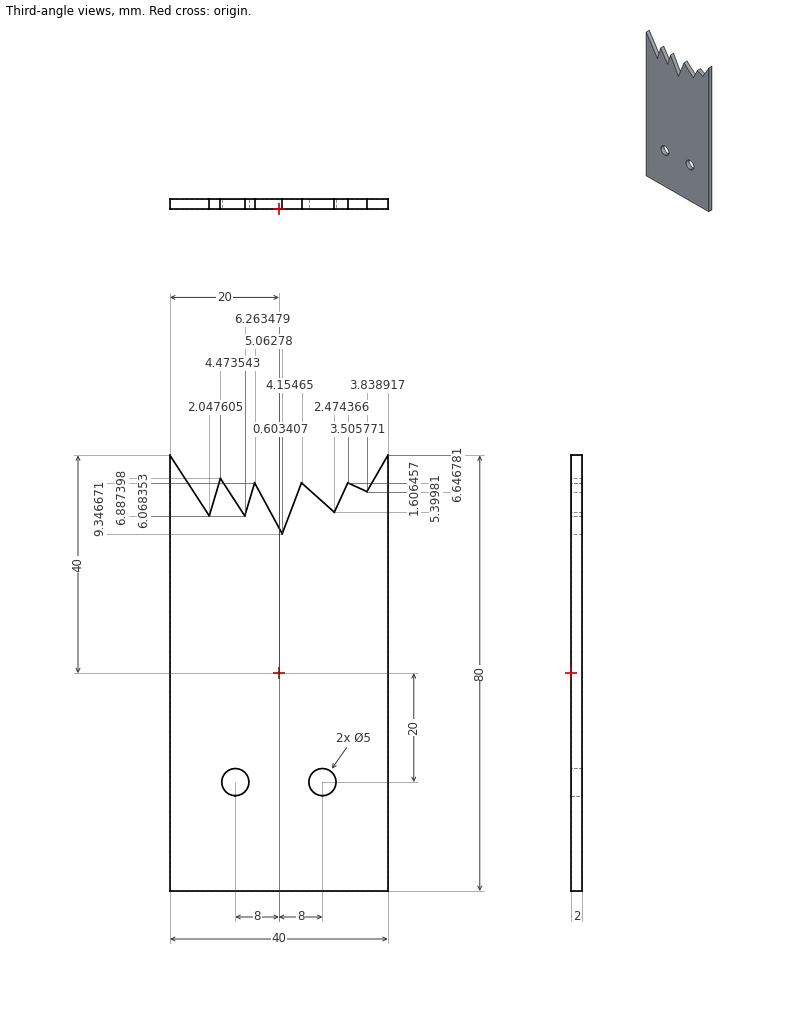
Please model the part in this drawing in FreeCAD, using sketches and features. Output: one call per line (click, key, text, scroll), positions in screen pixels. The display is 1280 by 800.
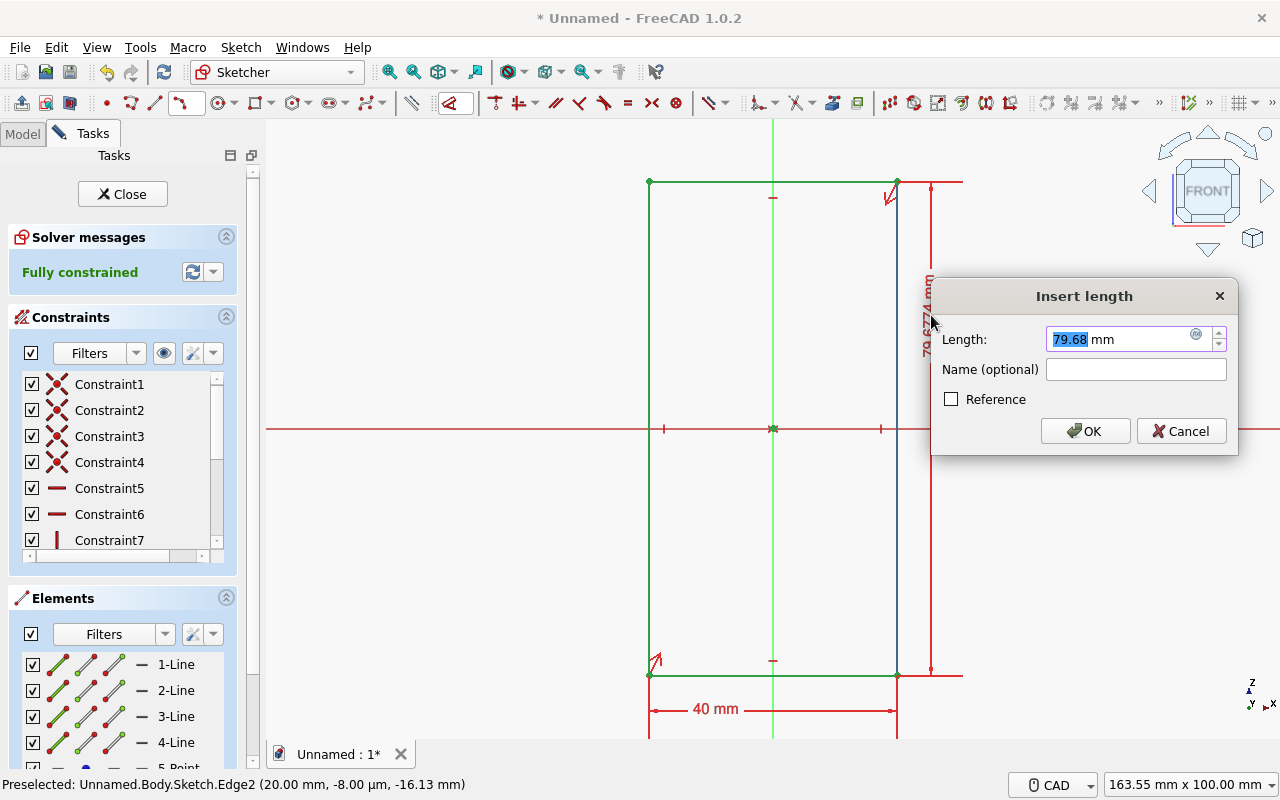
text(80)
key(Return)
key(Escape)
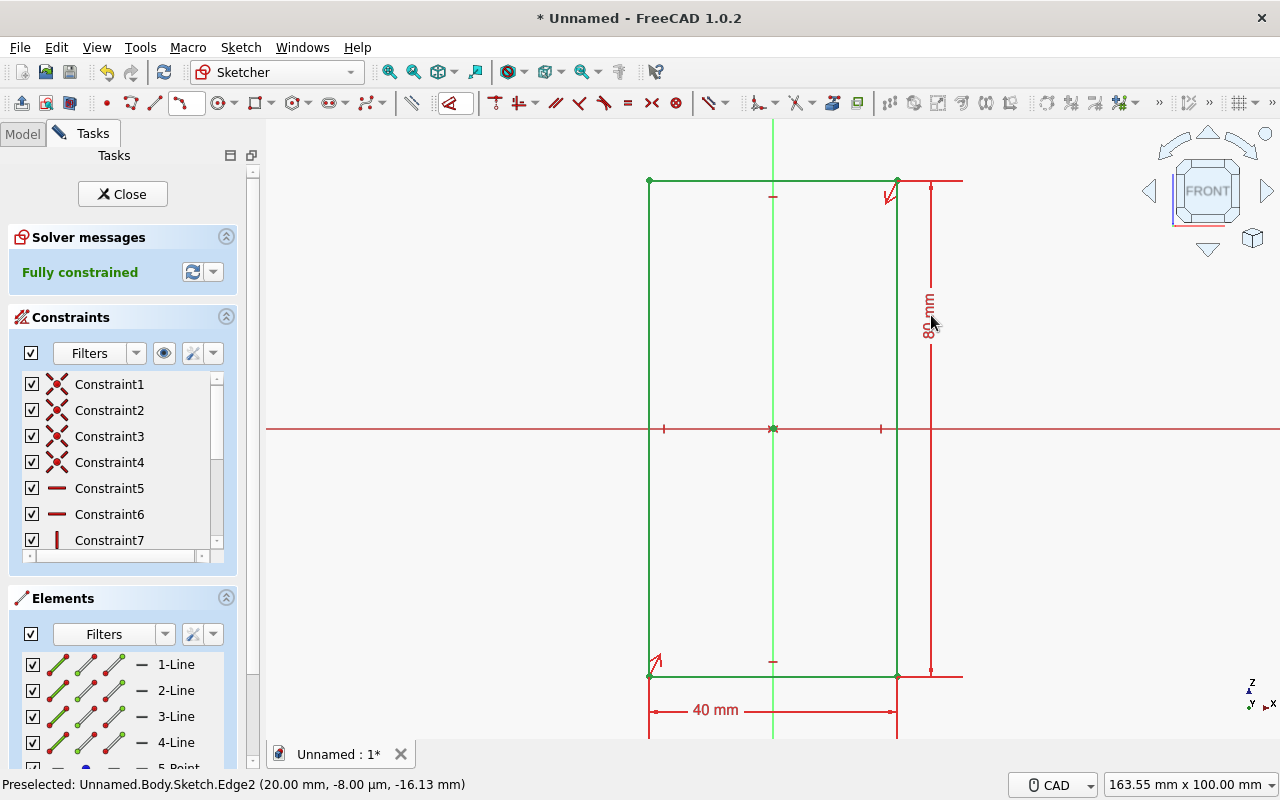
click(123, 194)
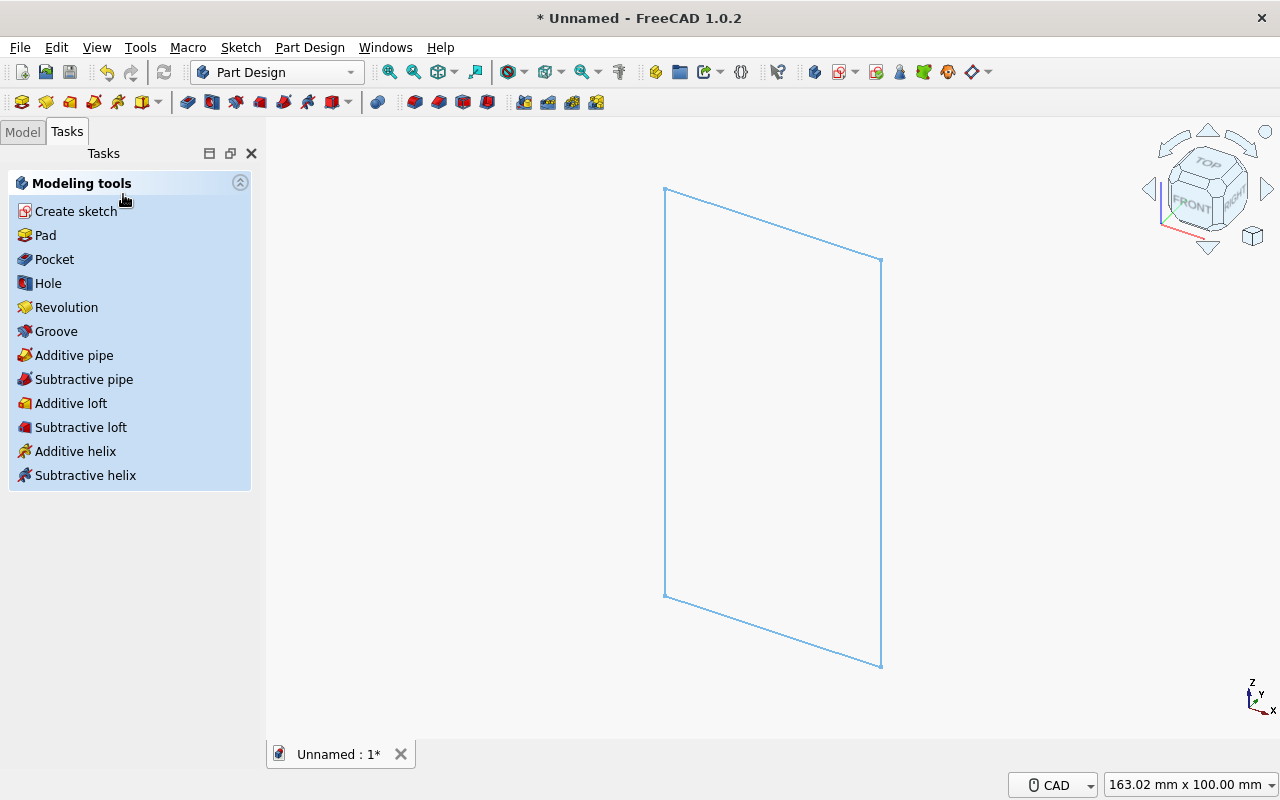
click(22, 102)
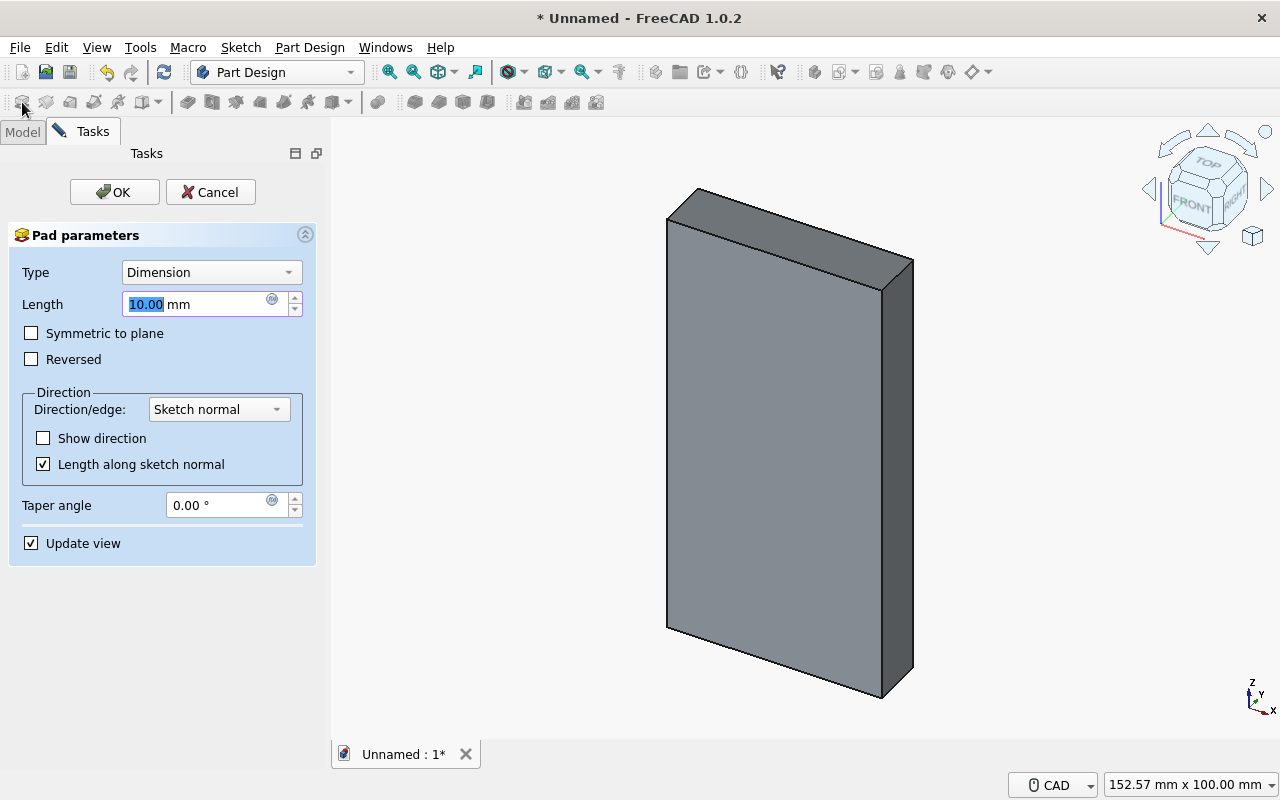
text(2)
key(Tab)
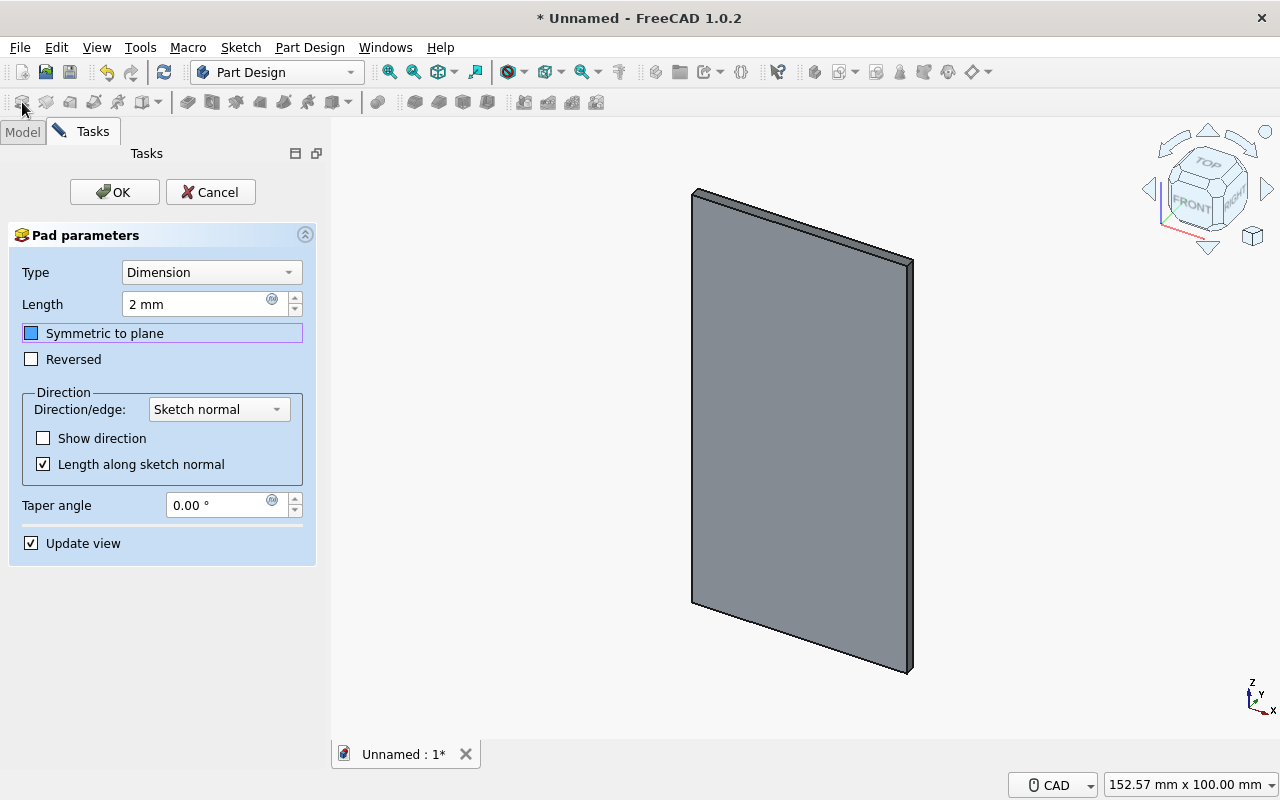
click(30, 359)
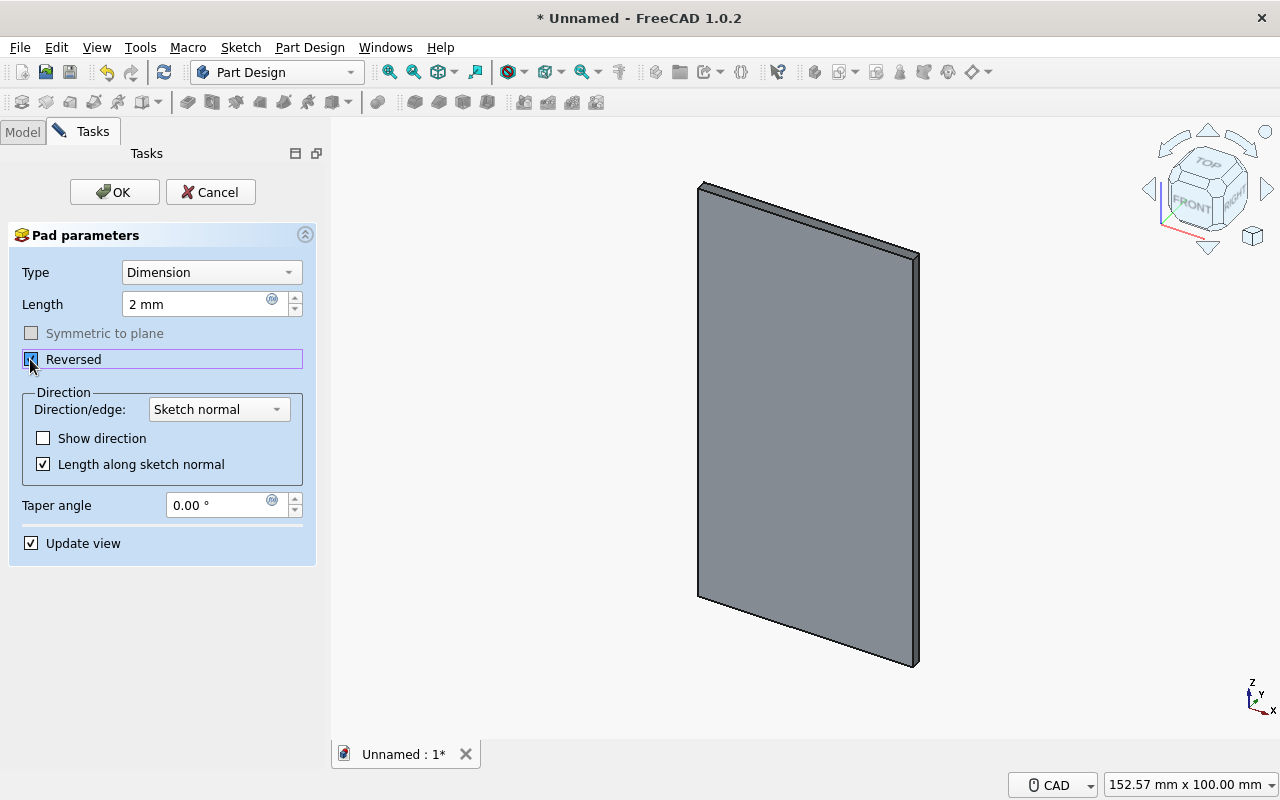
click(115, 192)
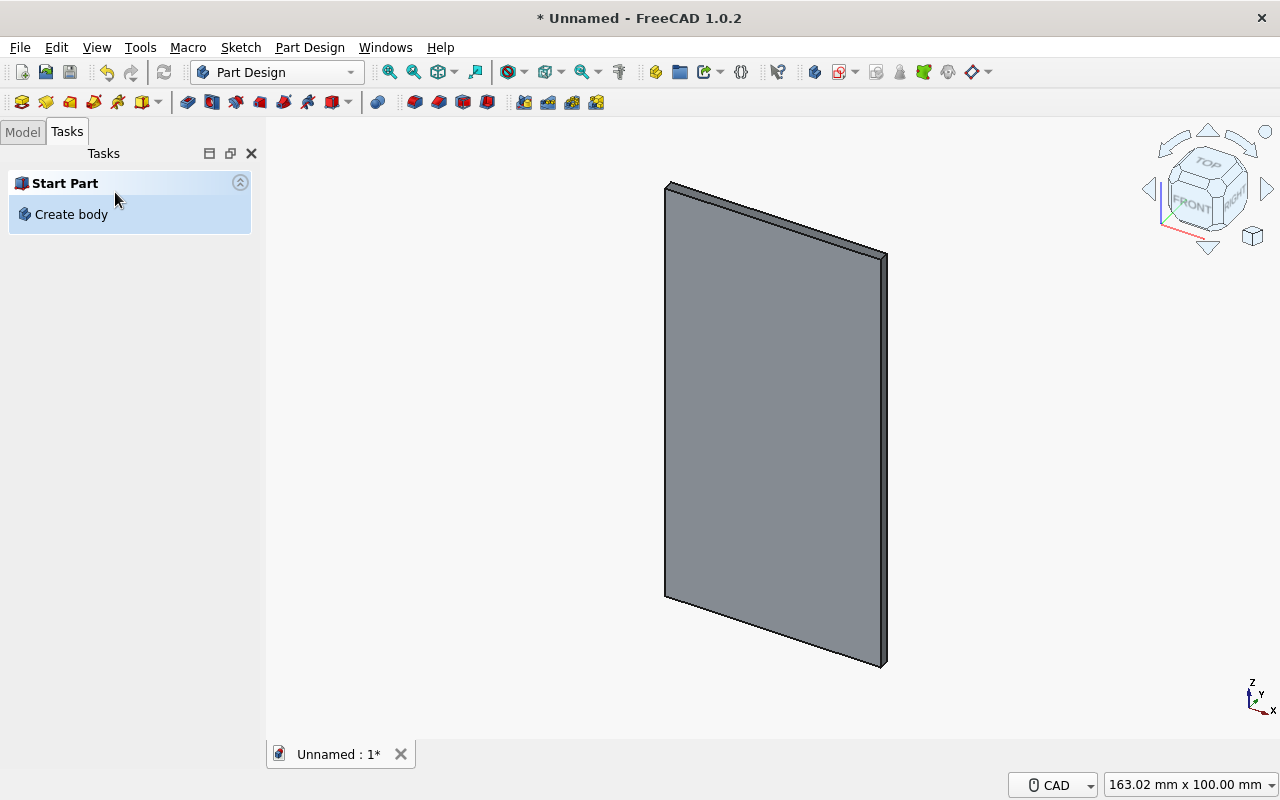
click(773, 369)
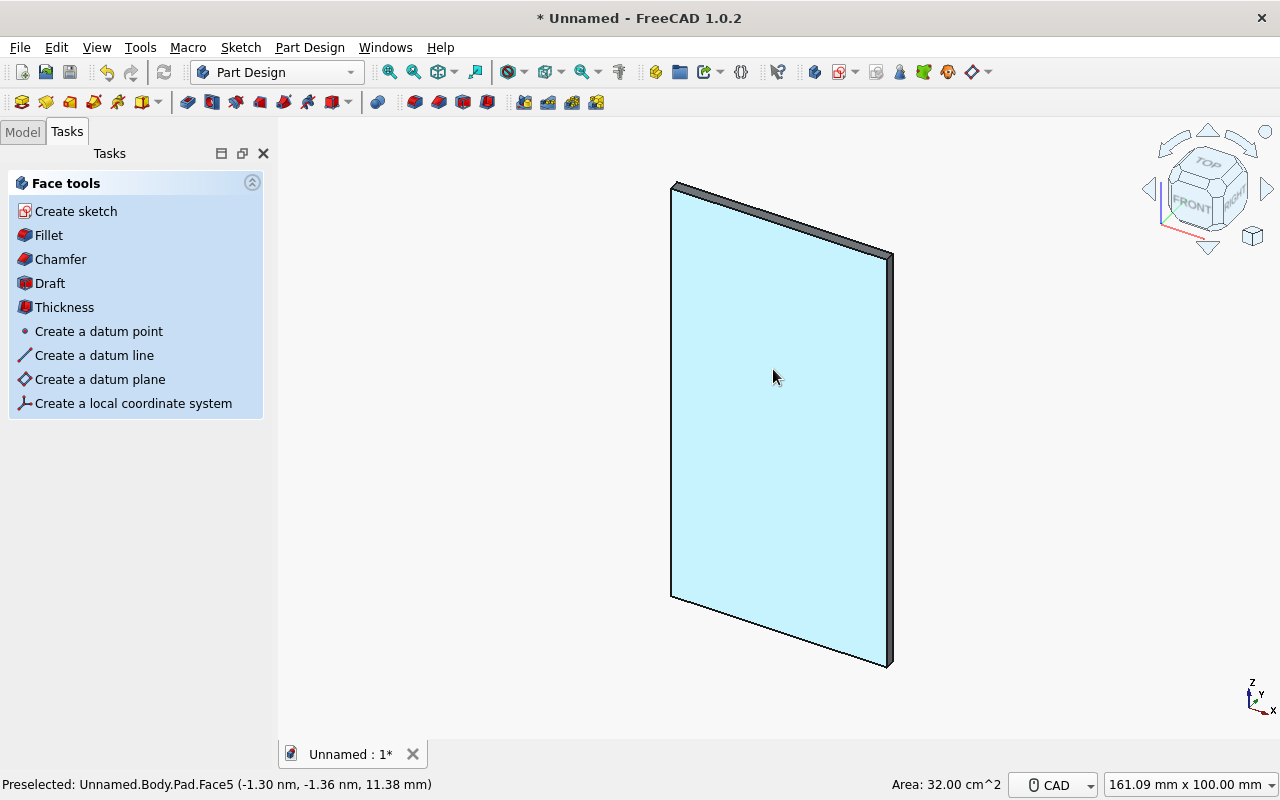
click(840, 72)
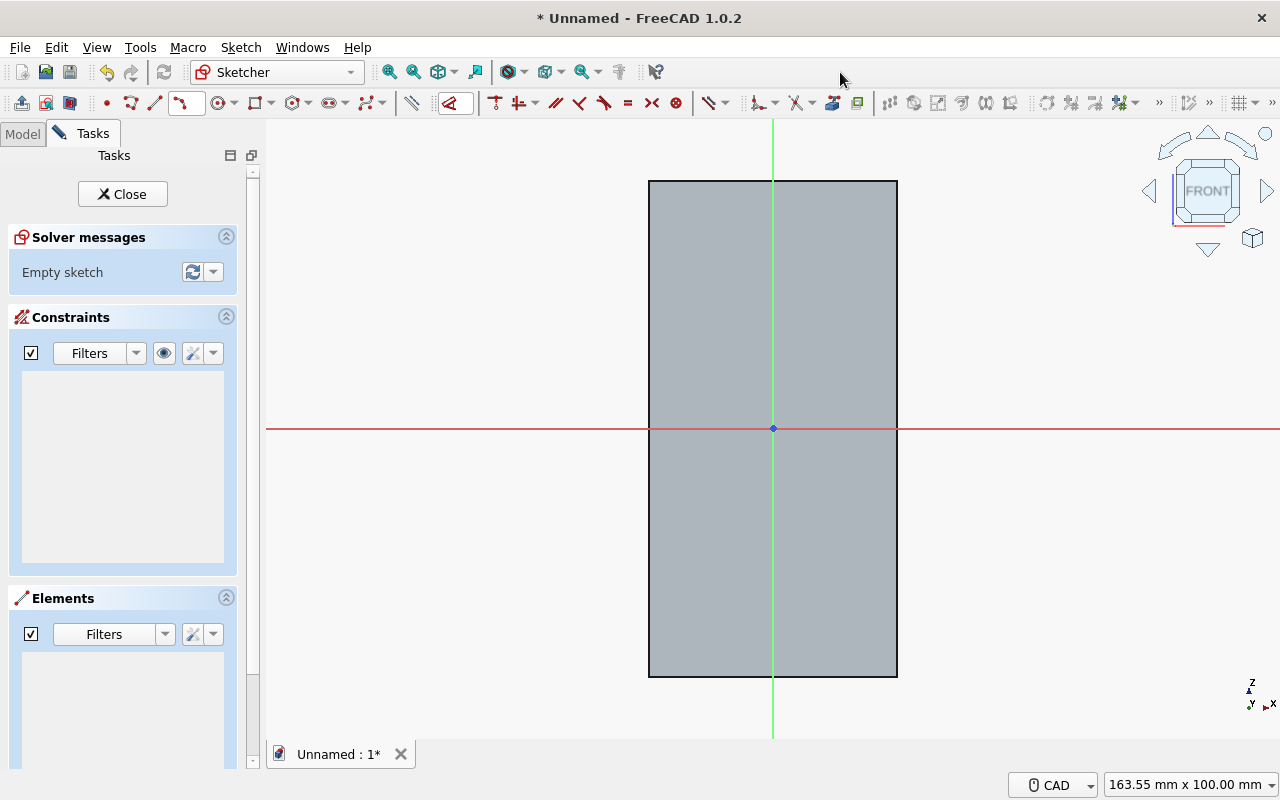
scroll(813, 539, up, 5)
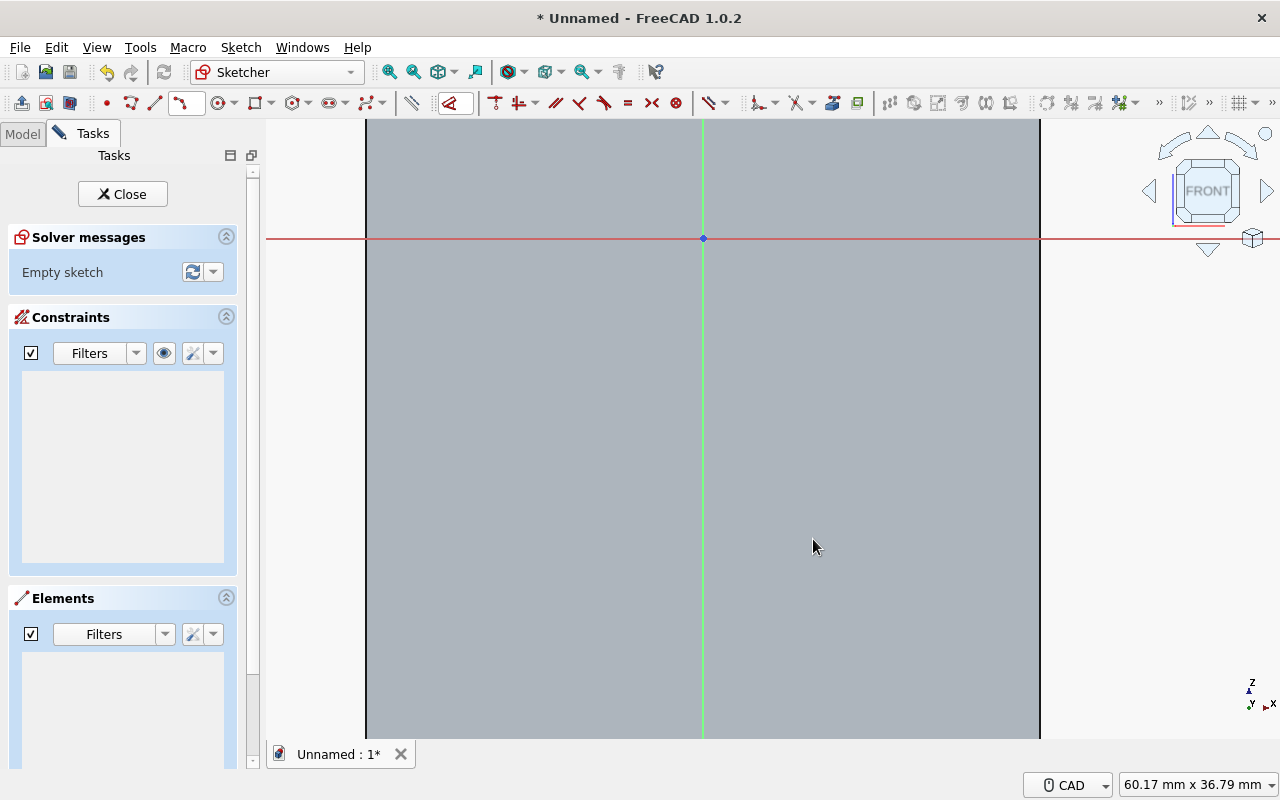
click(218, 104)